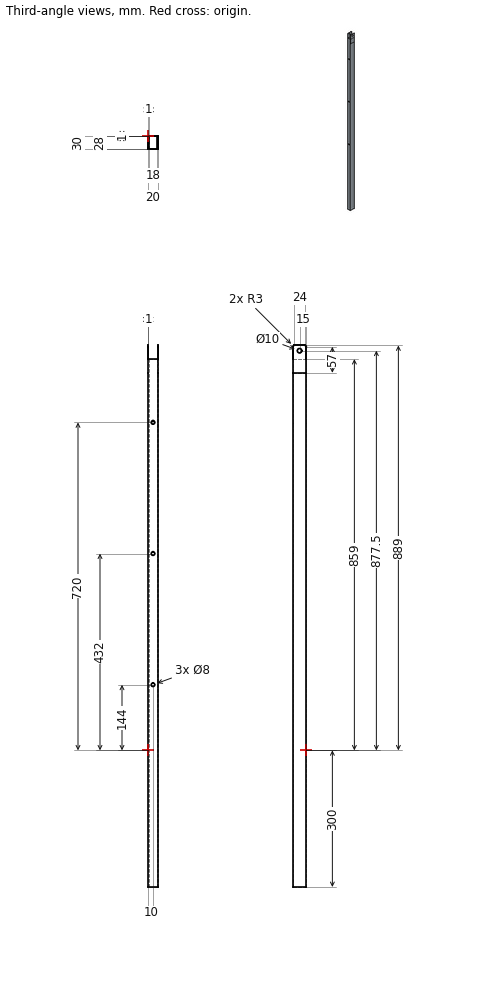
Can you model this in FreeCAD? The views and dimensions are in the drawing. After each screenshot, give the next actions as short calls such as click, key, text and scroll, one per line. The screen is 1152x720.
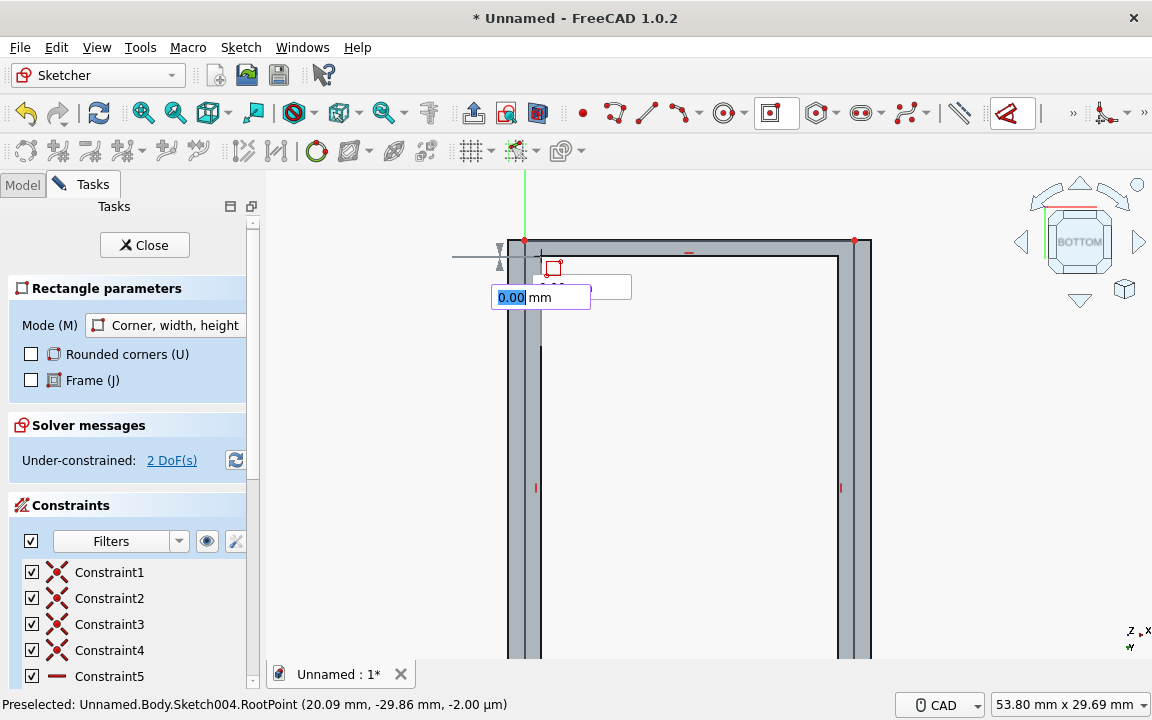
scroll(541, 268, down, 2)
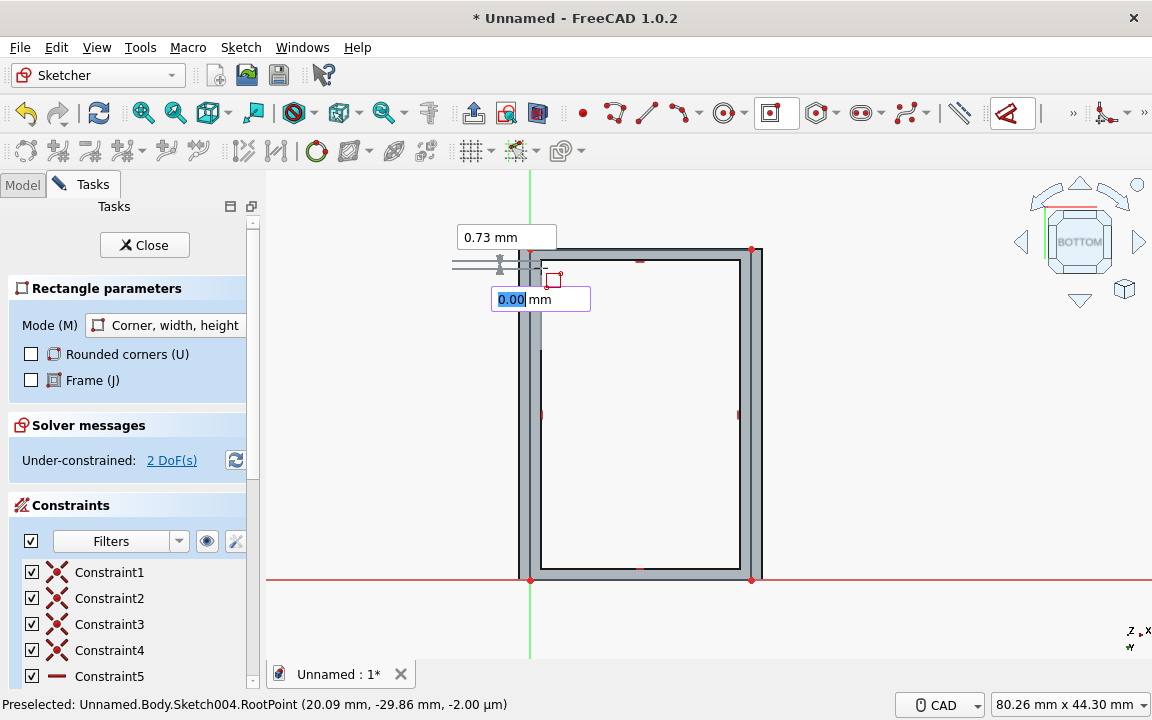
scroll(740, 569, up, 2)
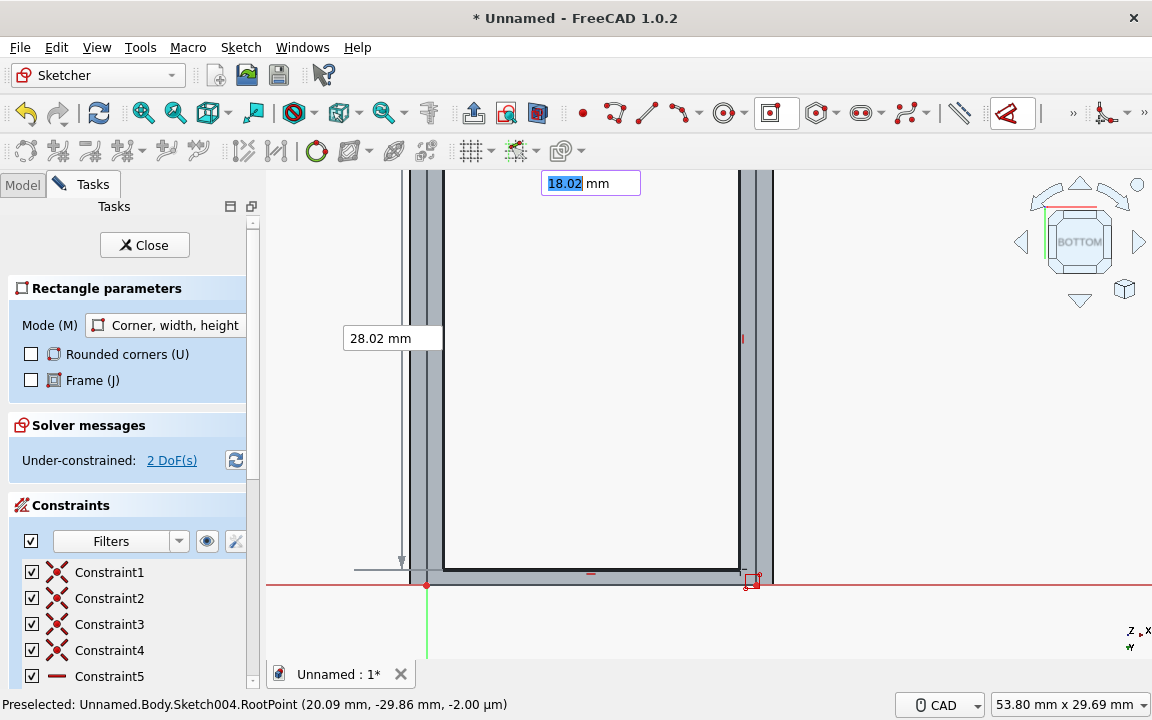
click(740, 569)
key(Escape)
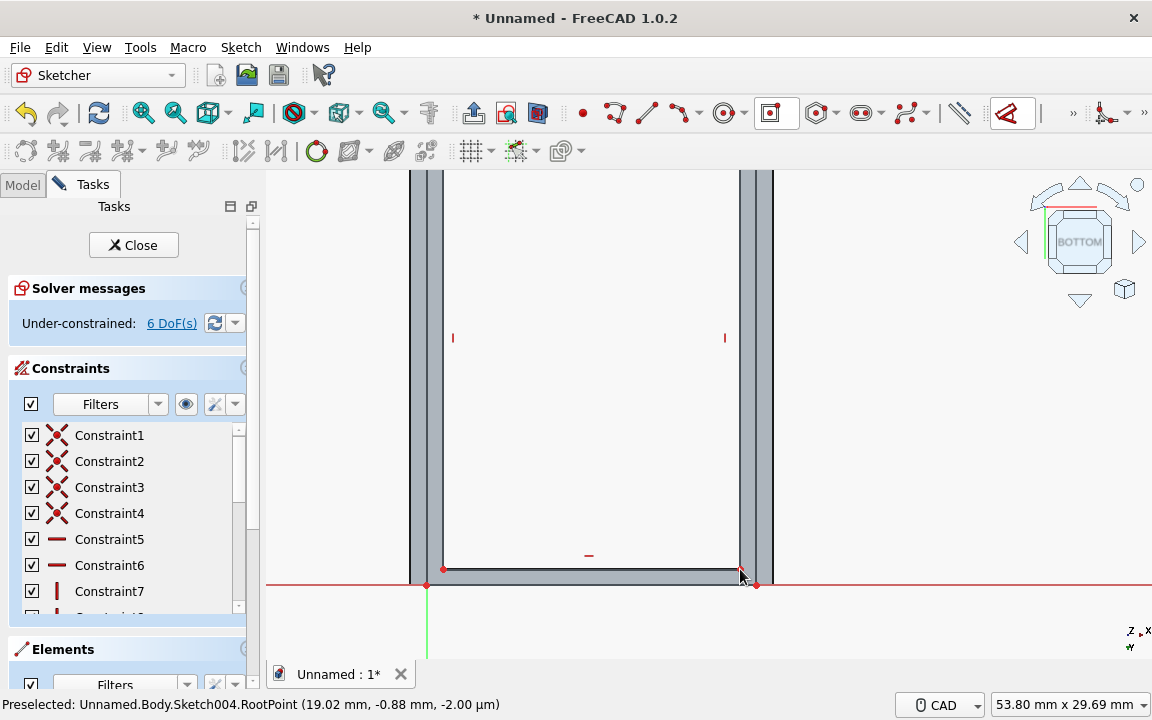
click(526, 585)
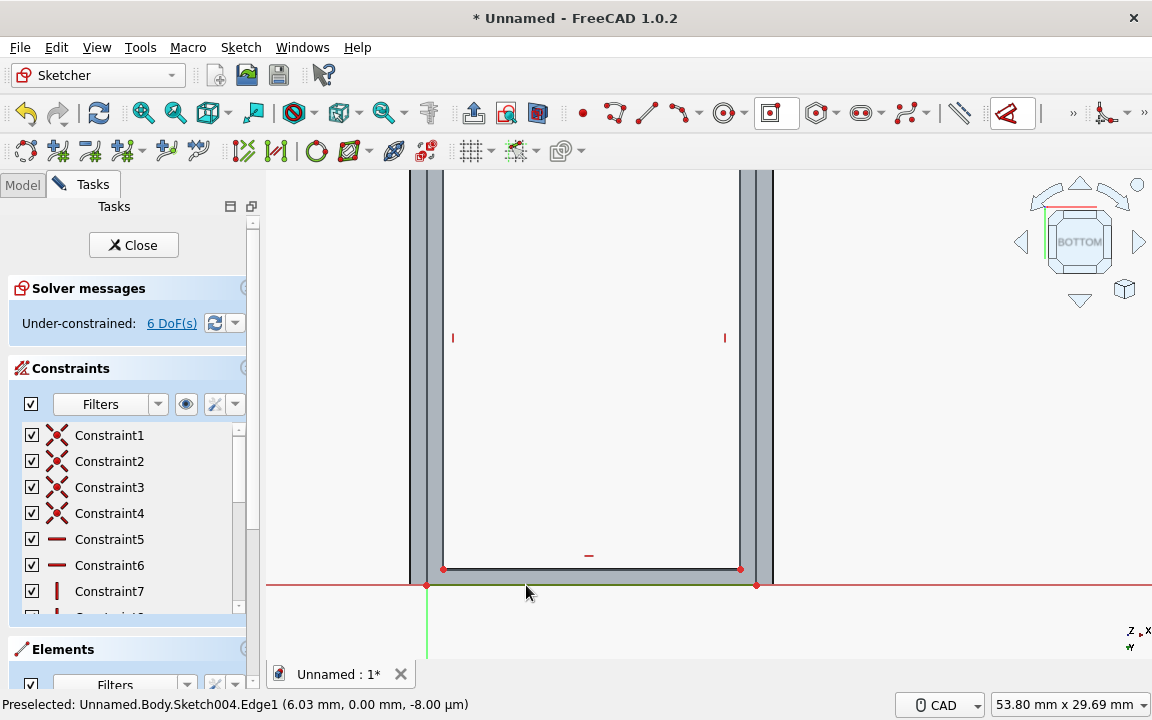
key(l)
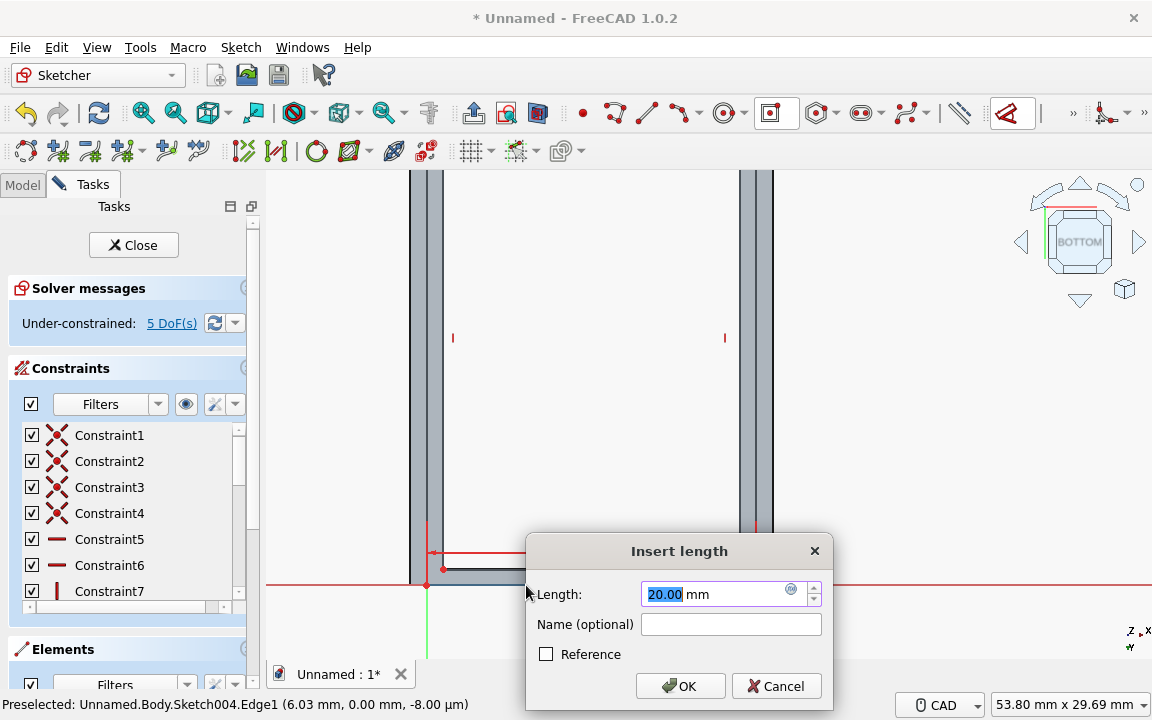
text(20)
key(Return)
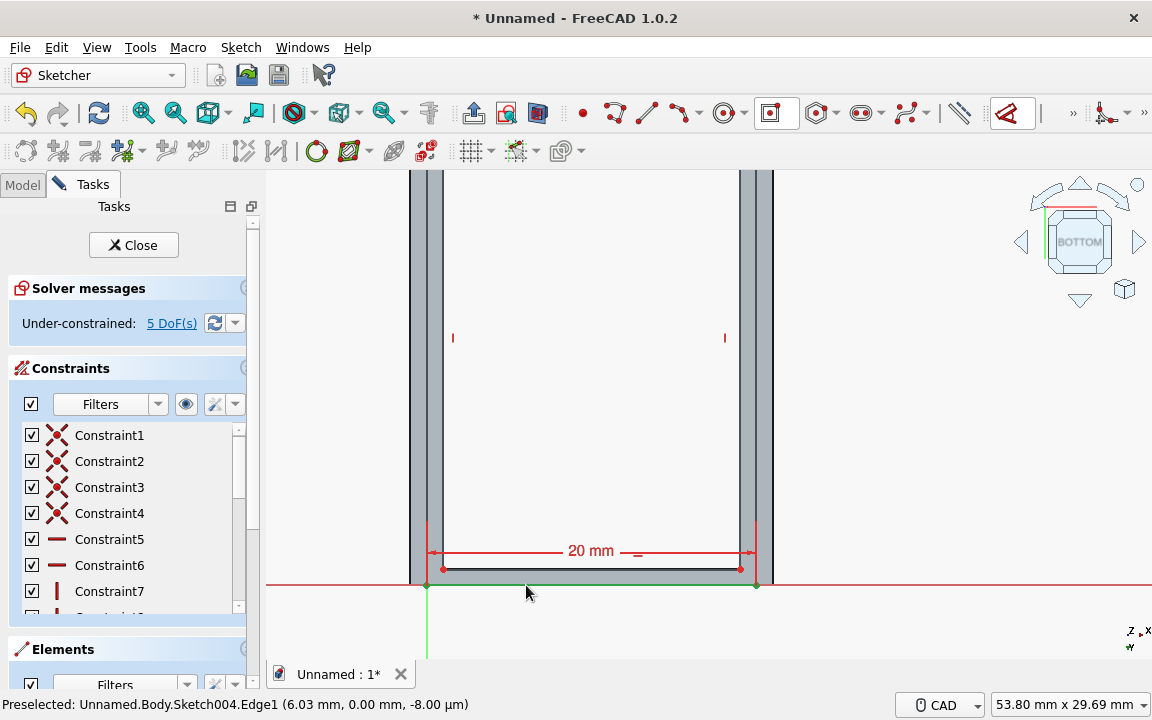
click(756, 437)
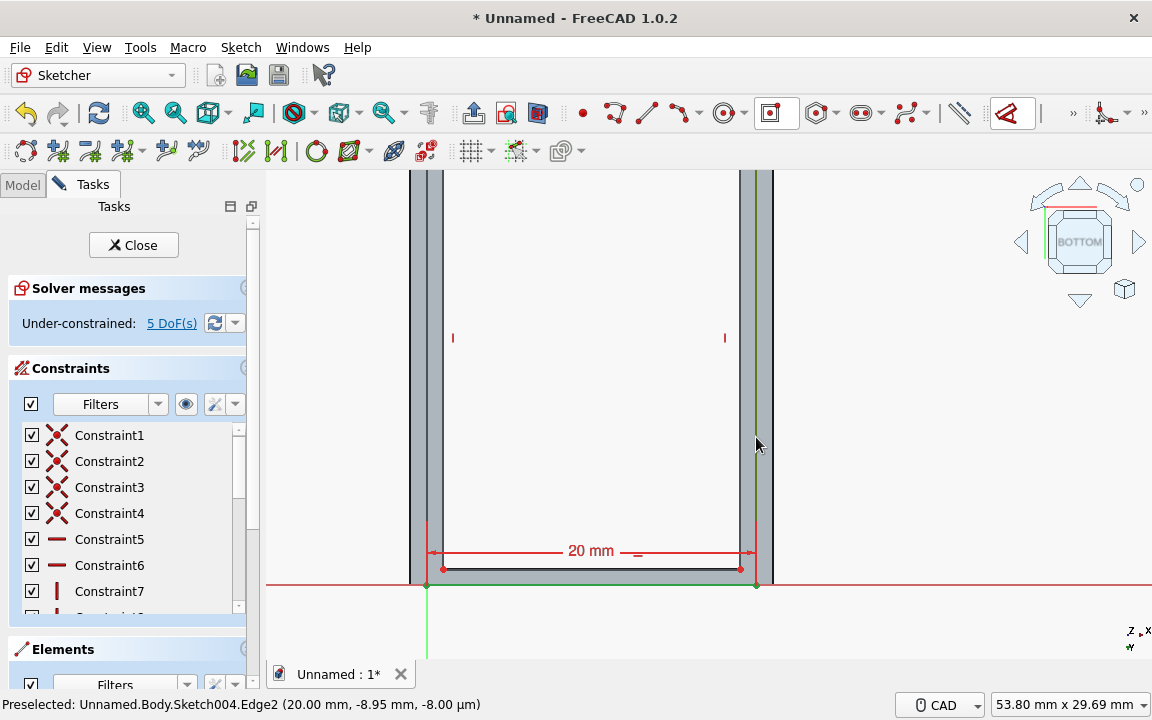
key(i)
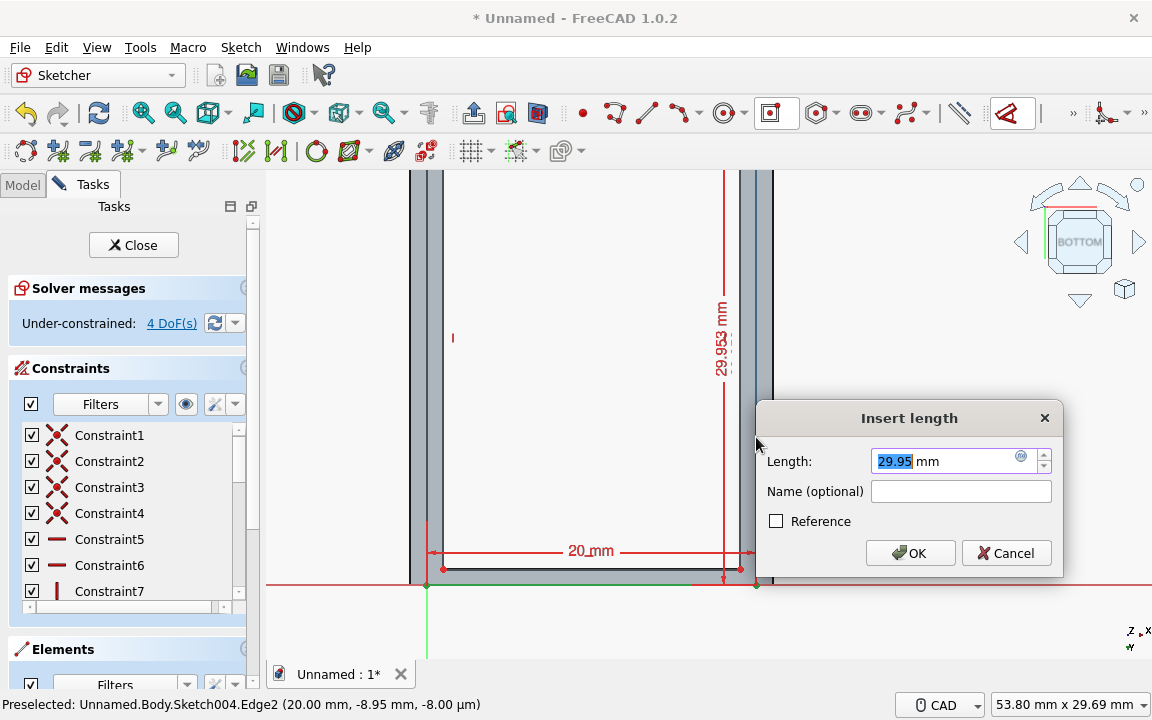
text(30)
key(Return)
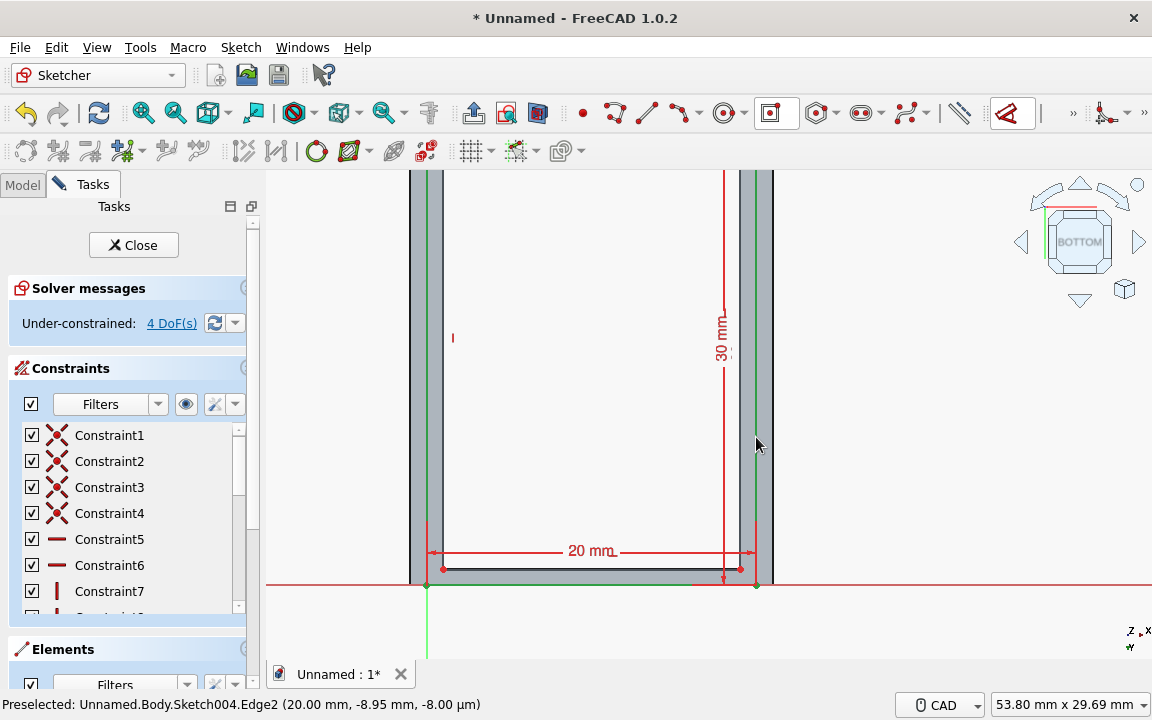
click(443, 247)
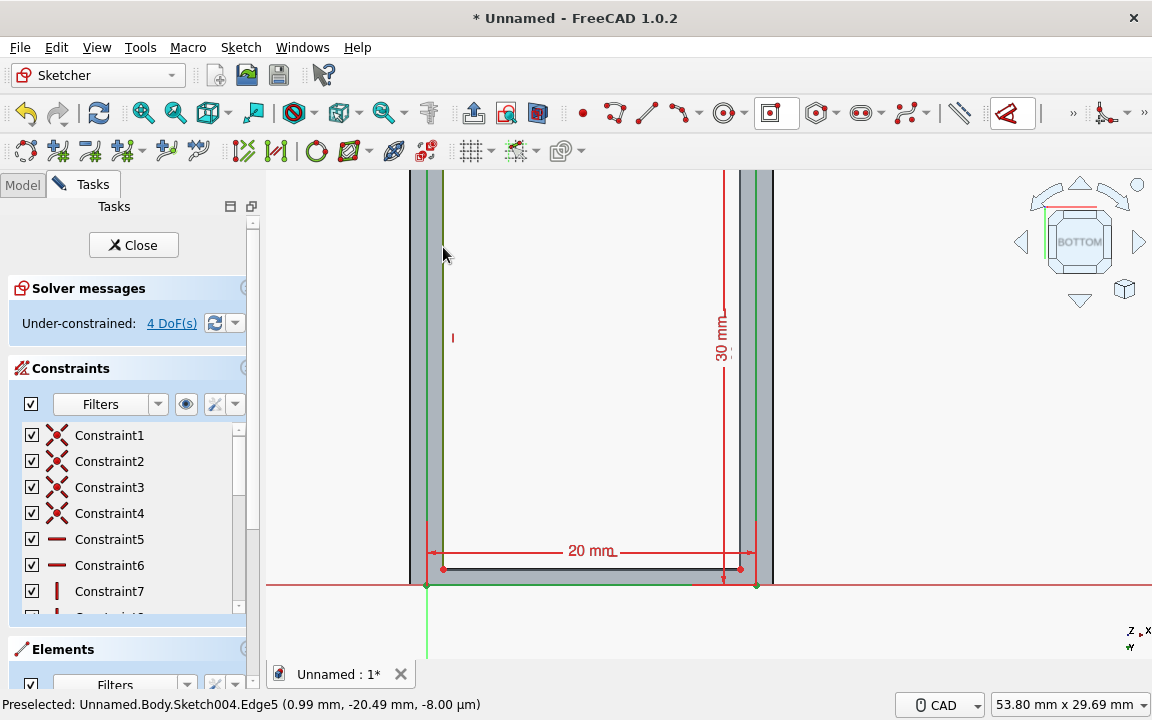
key(i)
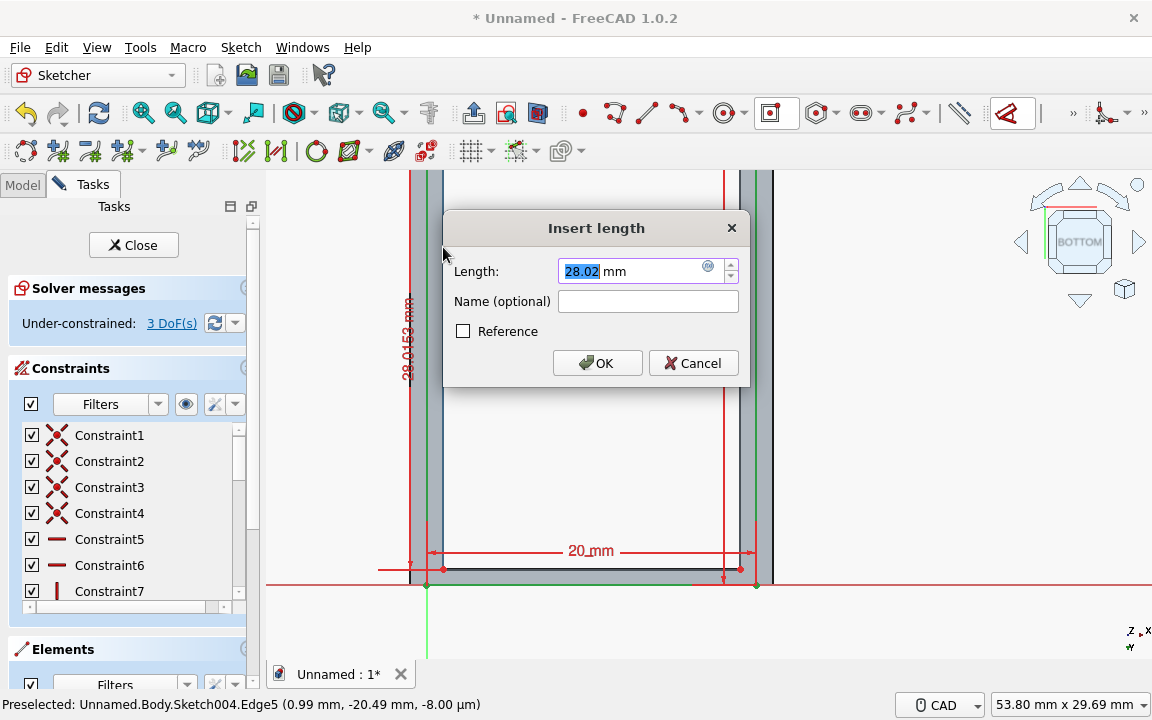
text(28)
key(Return)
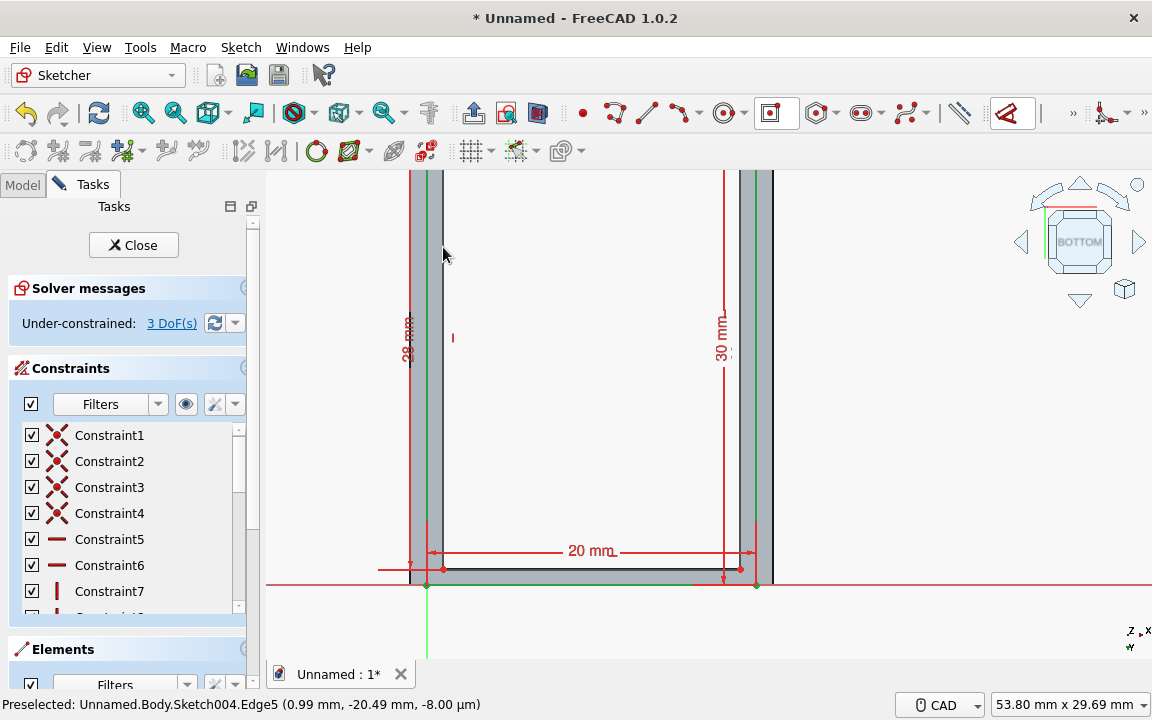
click(532, 570)